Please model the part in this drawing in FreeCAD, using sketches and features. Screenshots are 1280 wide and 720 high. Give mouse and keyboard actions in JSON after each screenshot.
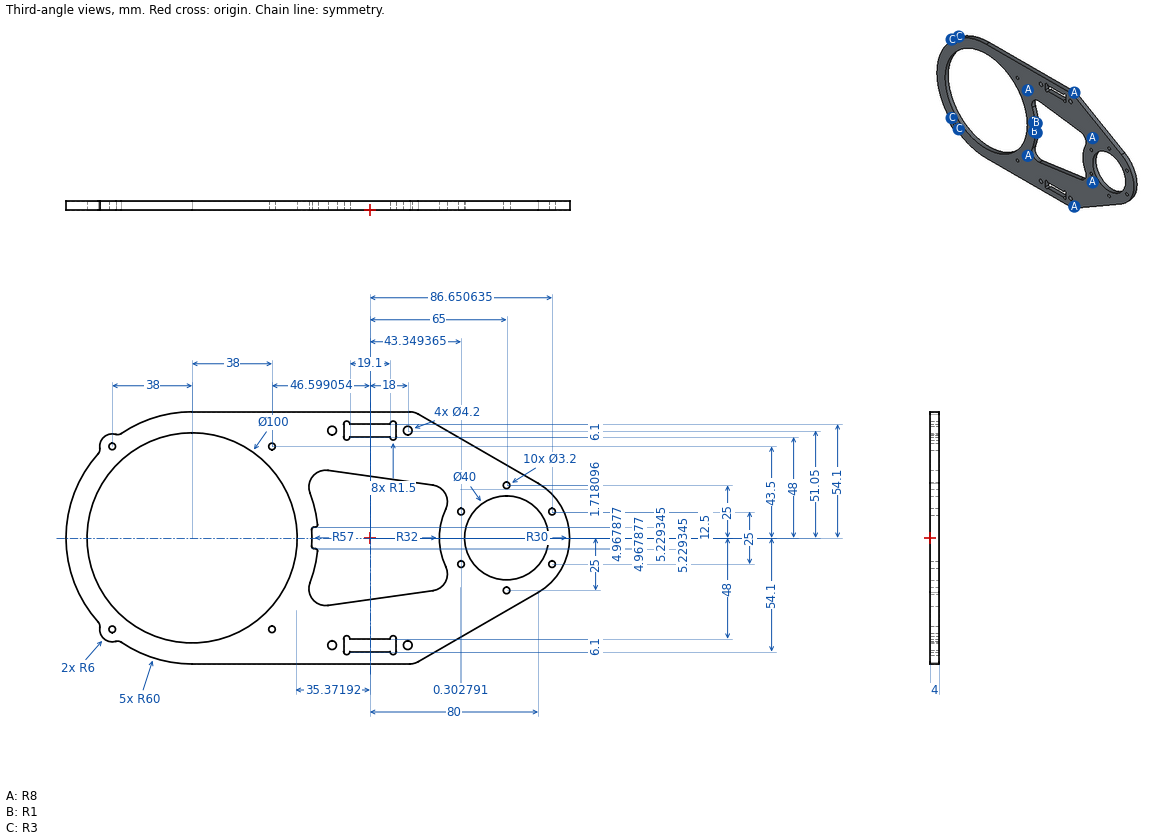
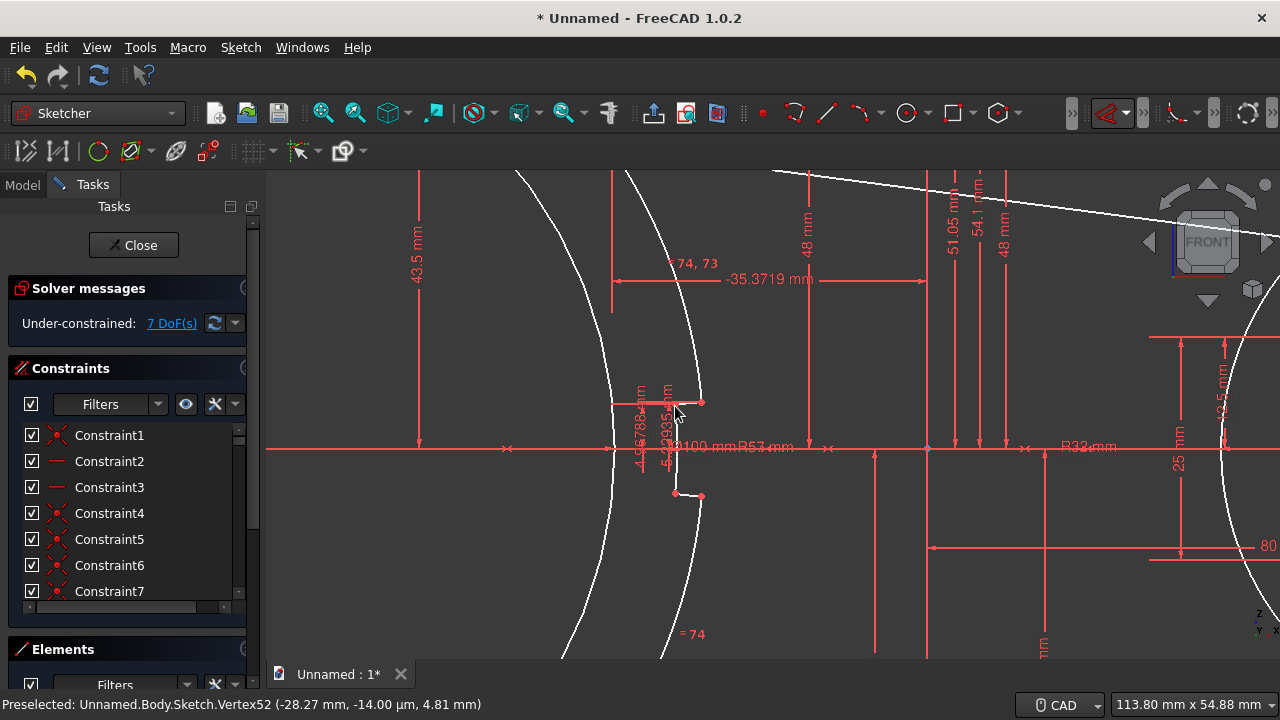
{"action": "left_click", "coordinate": [675, 494]}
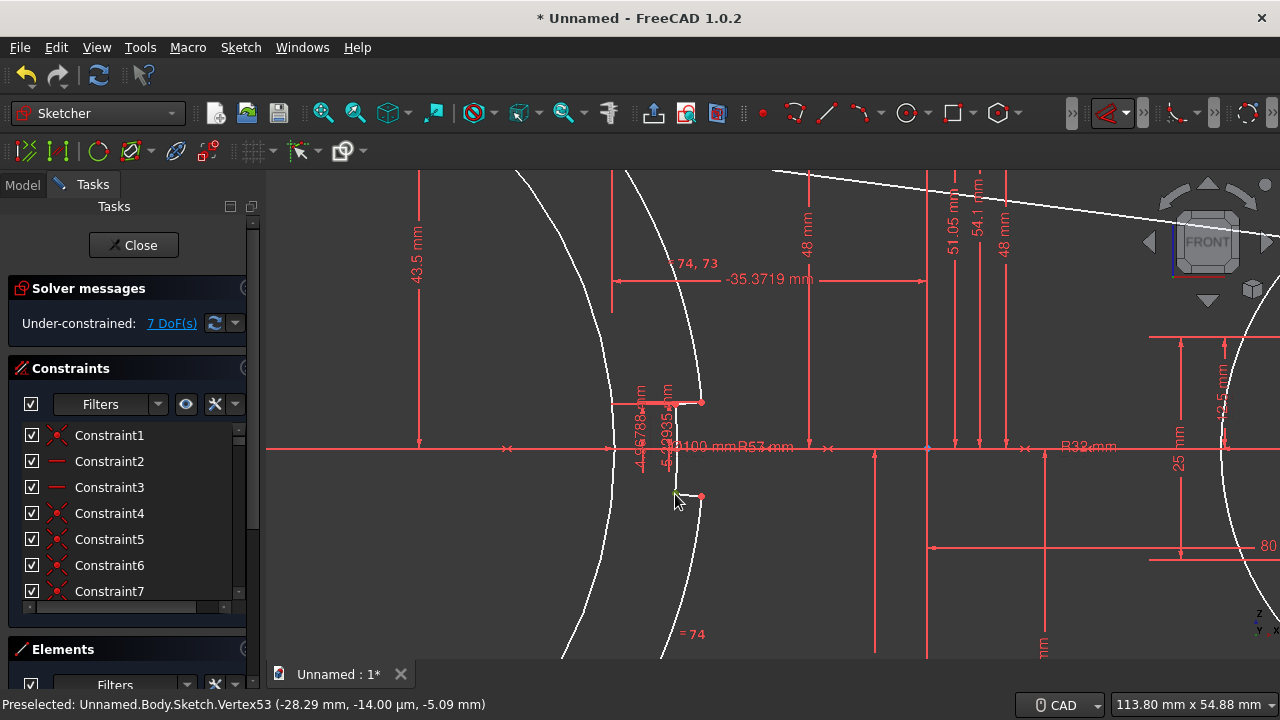
{"action": "left_click", "coordinate": [1128, 114]}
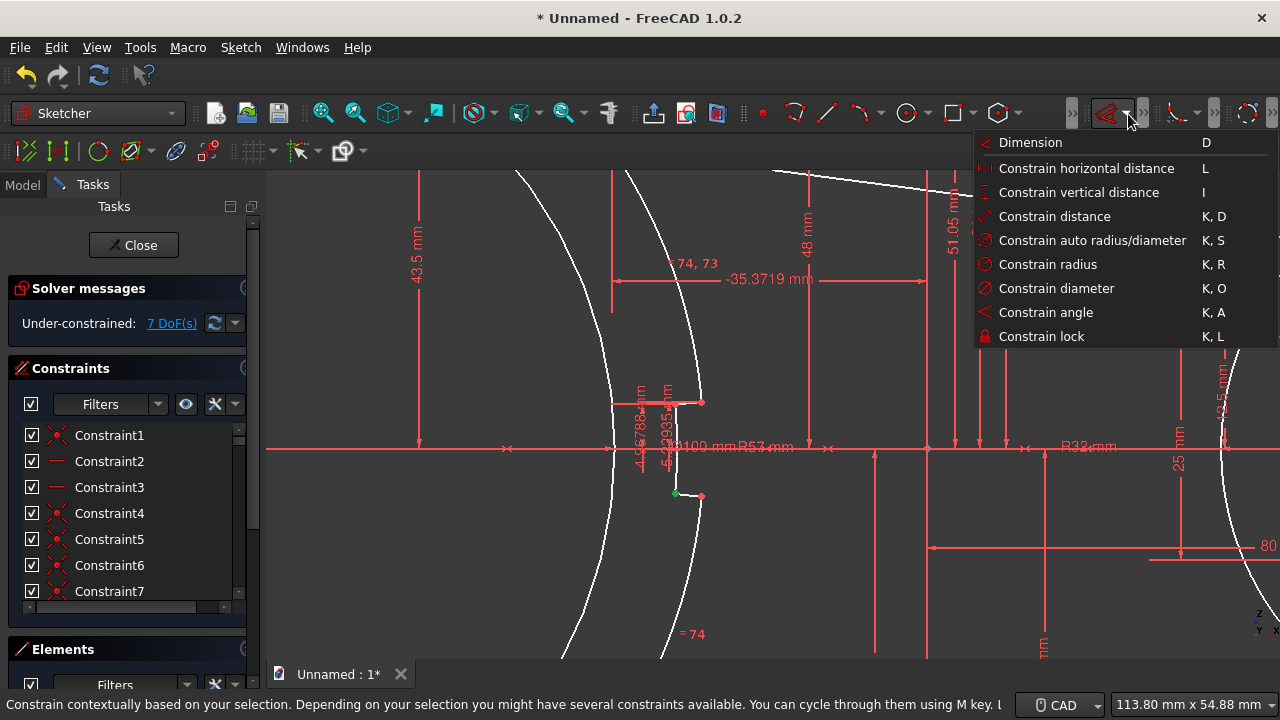
{"action": "left_click", "coordinate": [1126, 192]}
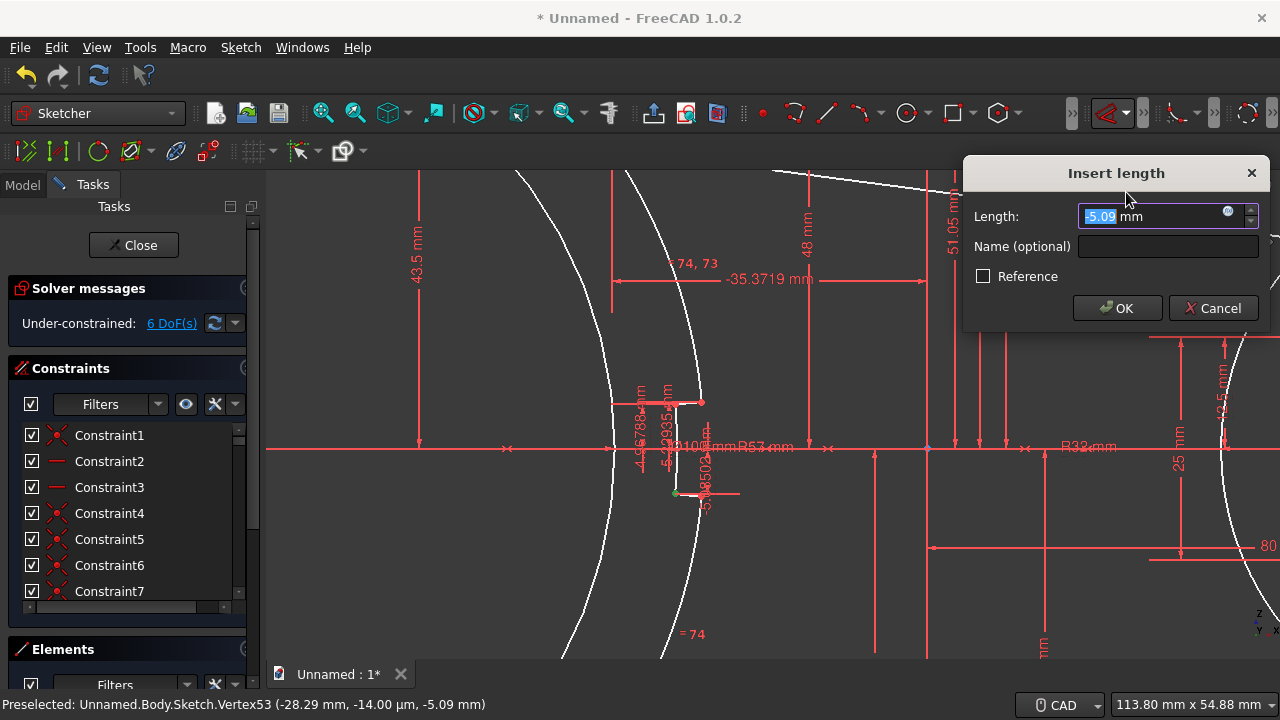
{"action": "type", "text": "-4.967877"}
{"action": "key", "text": "Return"}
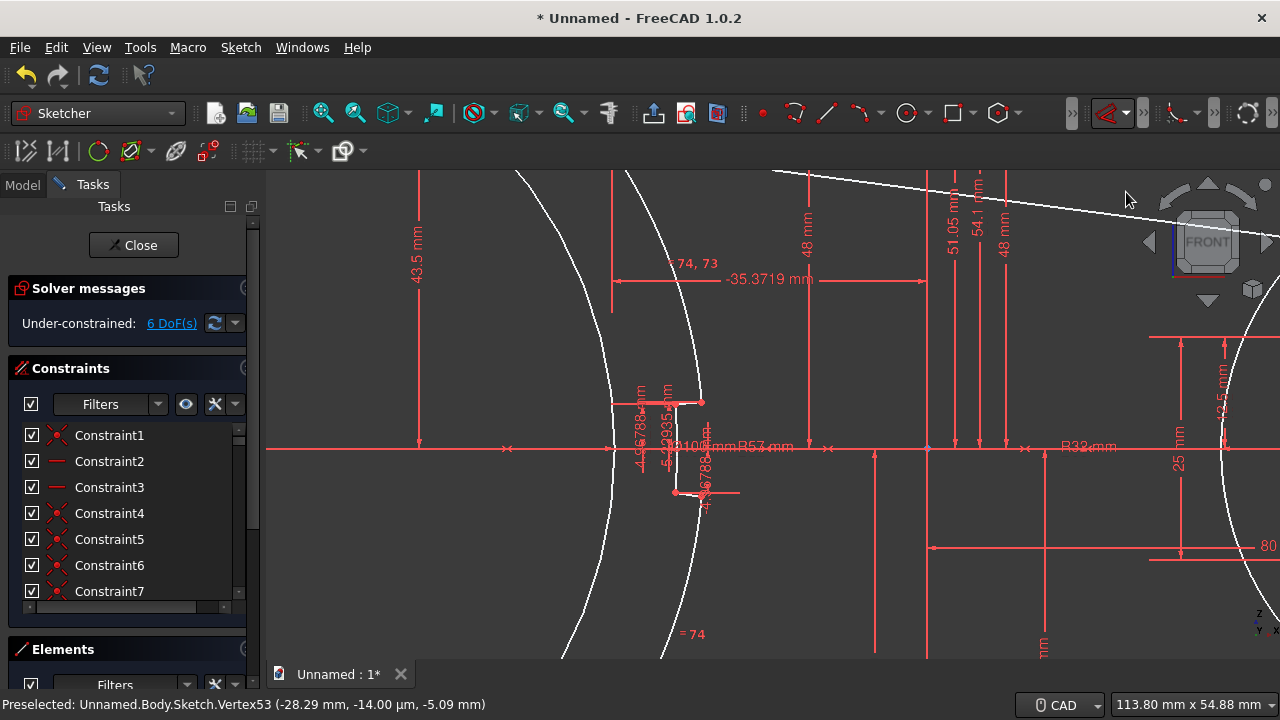
{"action": "left_click", "coordinate": [702, 497]}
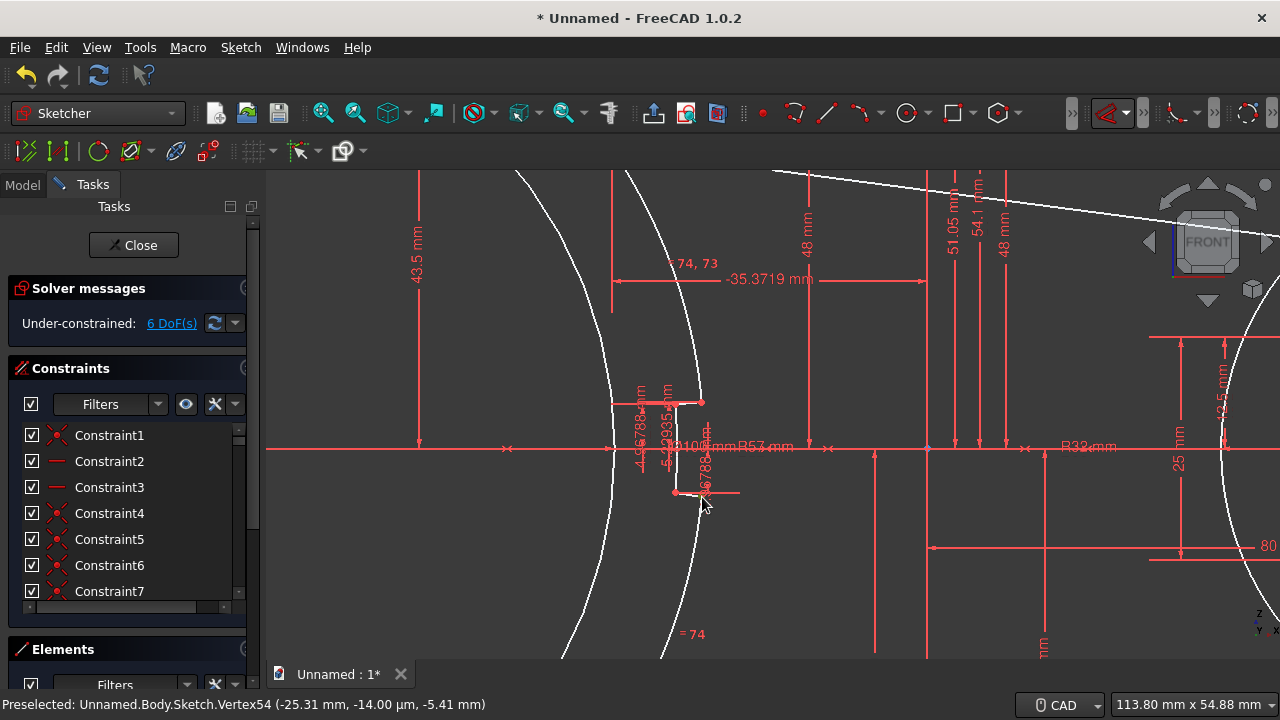
{"action": "left_click", "coordinate": [1128, 114]}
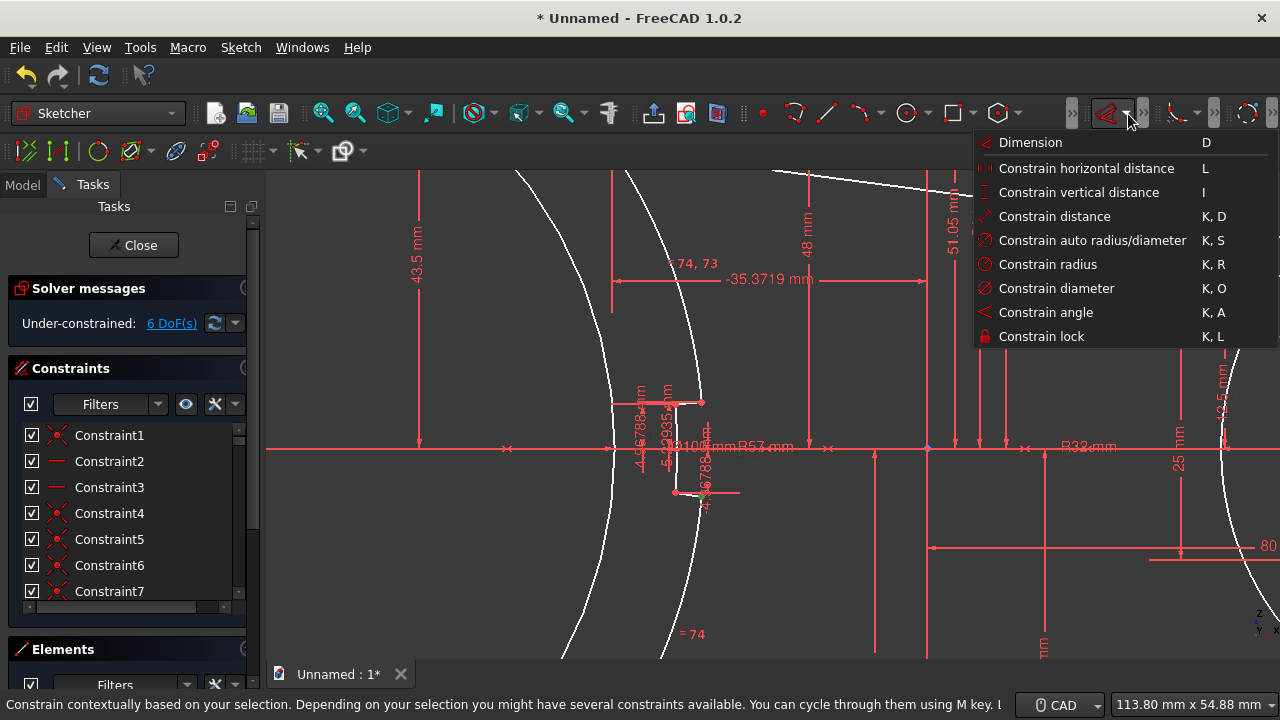
{"action": "left_click", "coordinate": [1126, 192]}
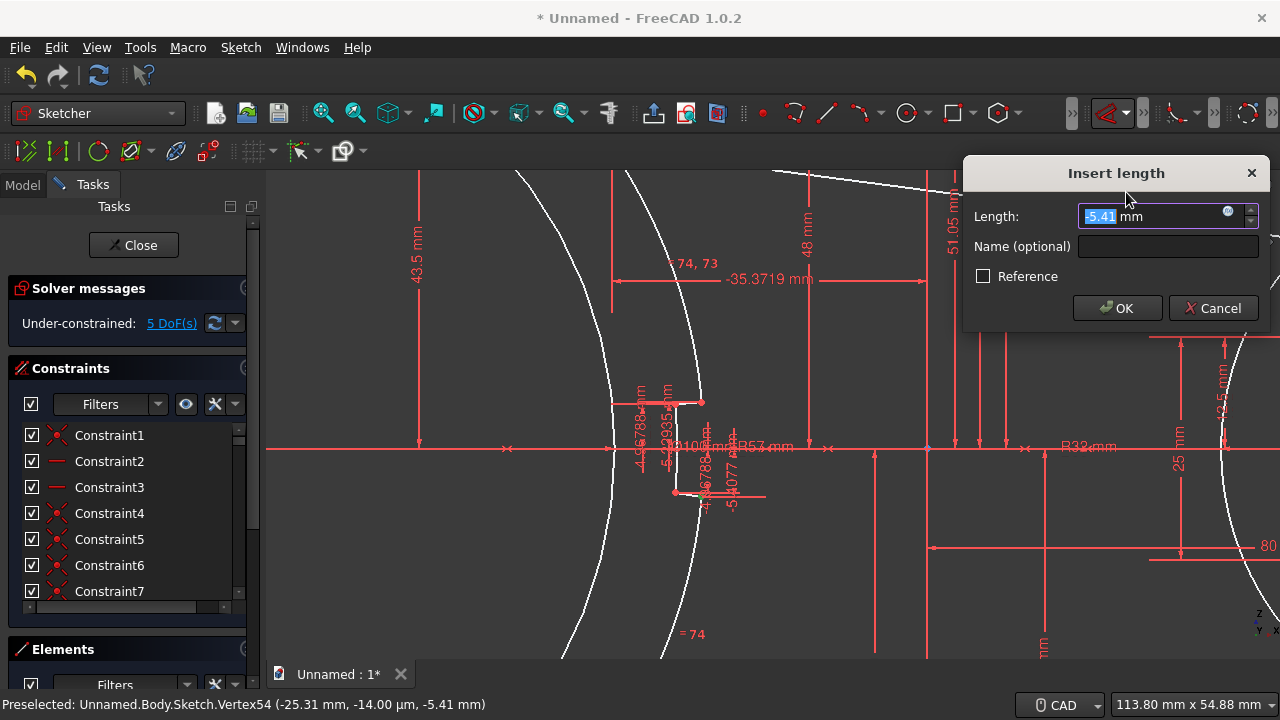
{"action": "type", "text": "-5.229345"}
{"action": "key", "text": "Return"}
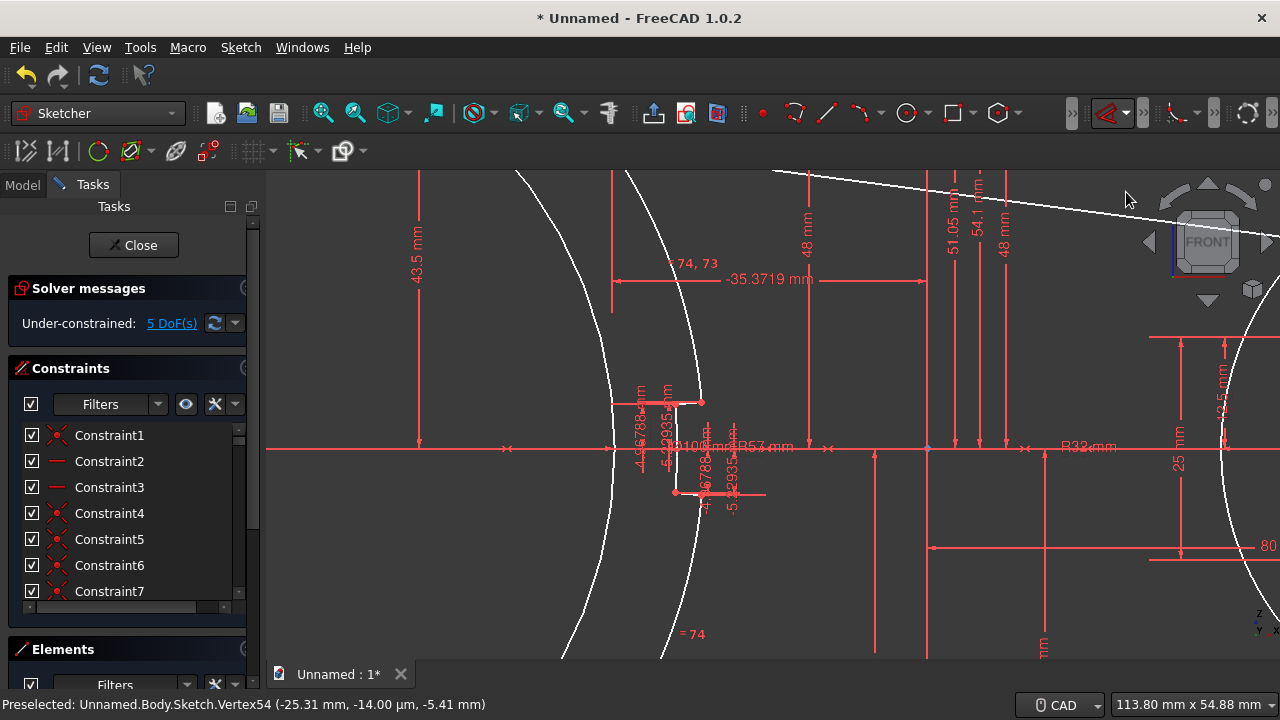
{"action": "scroll", "coordinate": [704, 403], "scroll_direction": "down", "scroll_amount": 7}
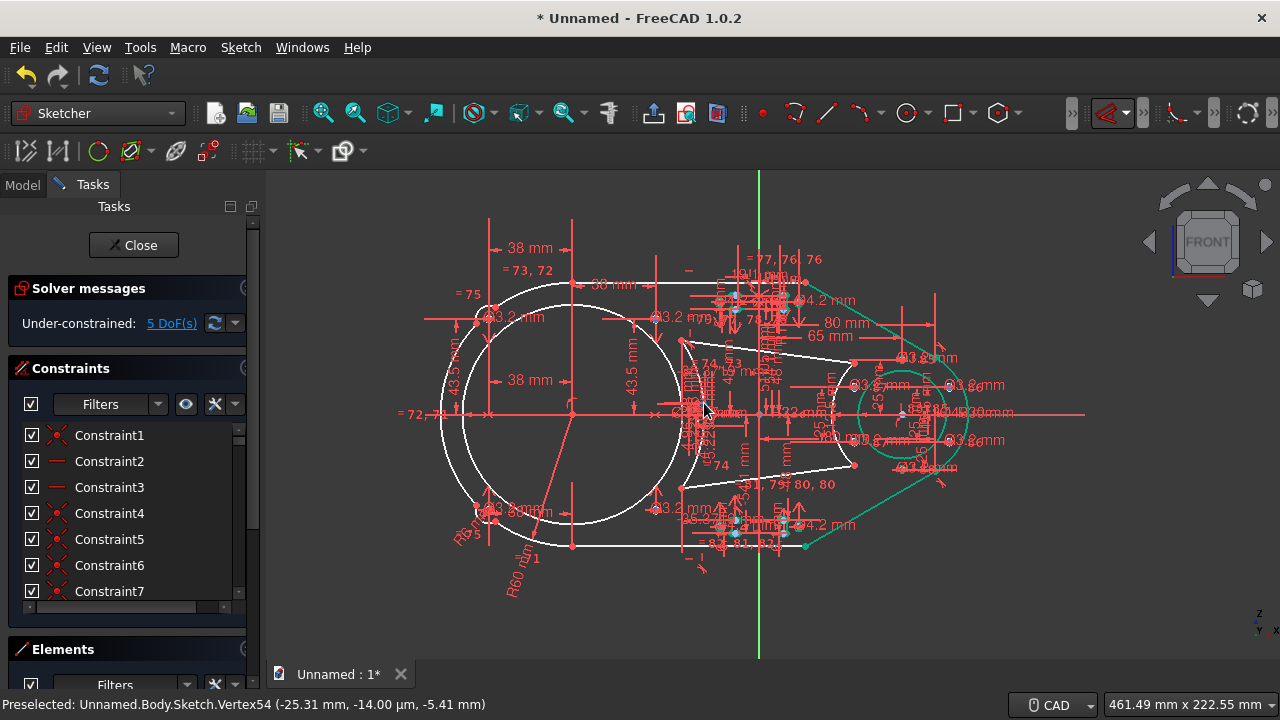
{"action": "left_click", "coordinate": [950, 387]}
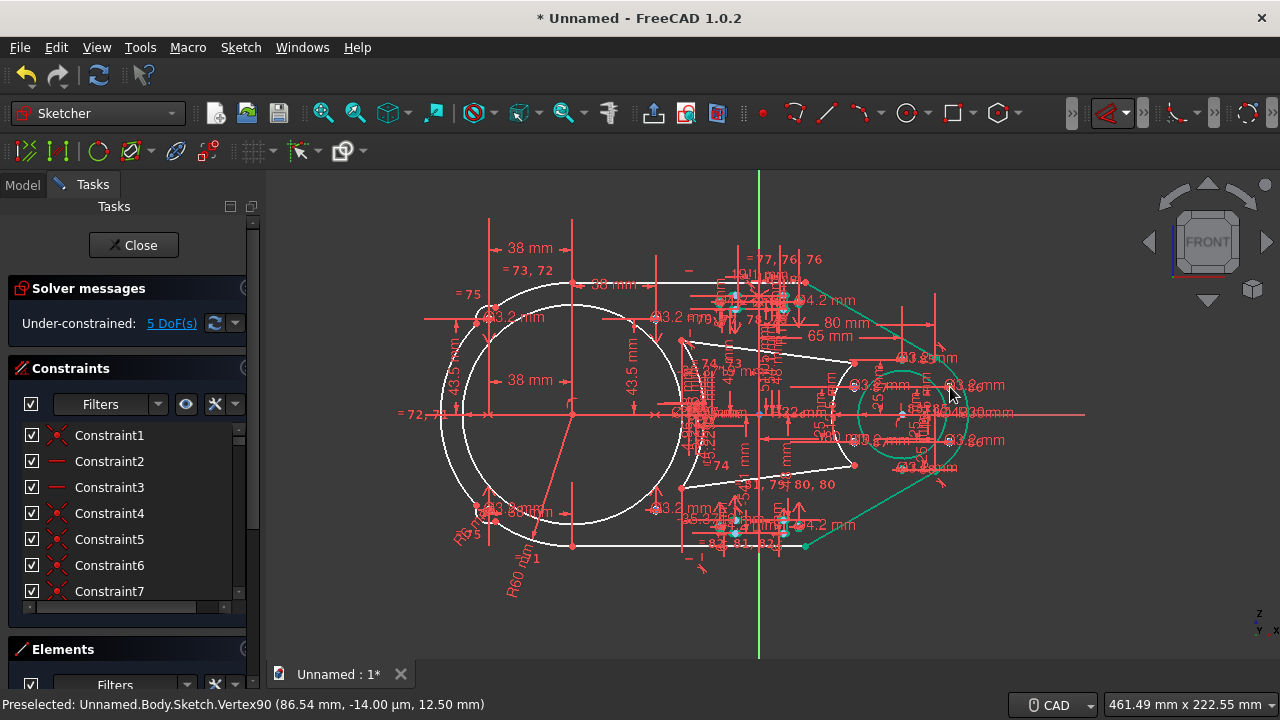
{"action": "key", "text": "l"}